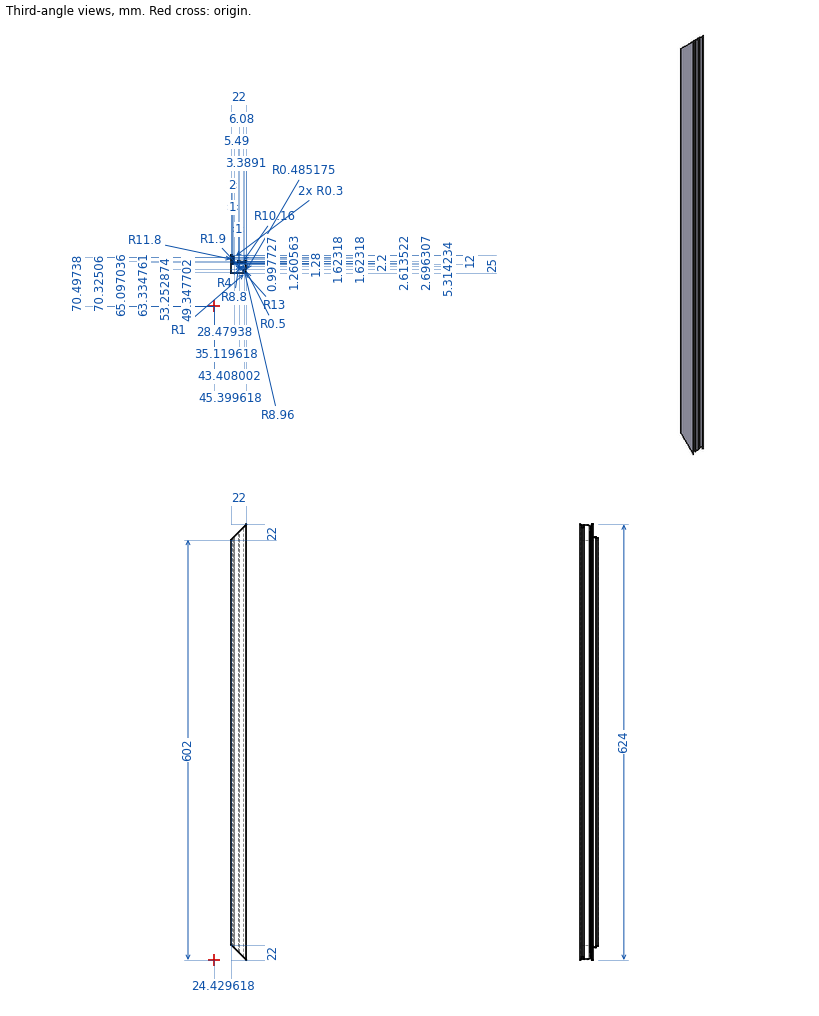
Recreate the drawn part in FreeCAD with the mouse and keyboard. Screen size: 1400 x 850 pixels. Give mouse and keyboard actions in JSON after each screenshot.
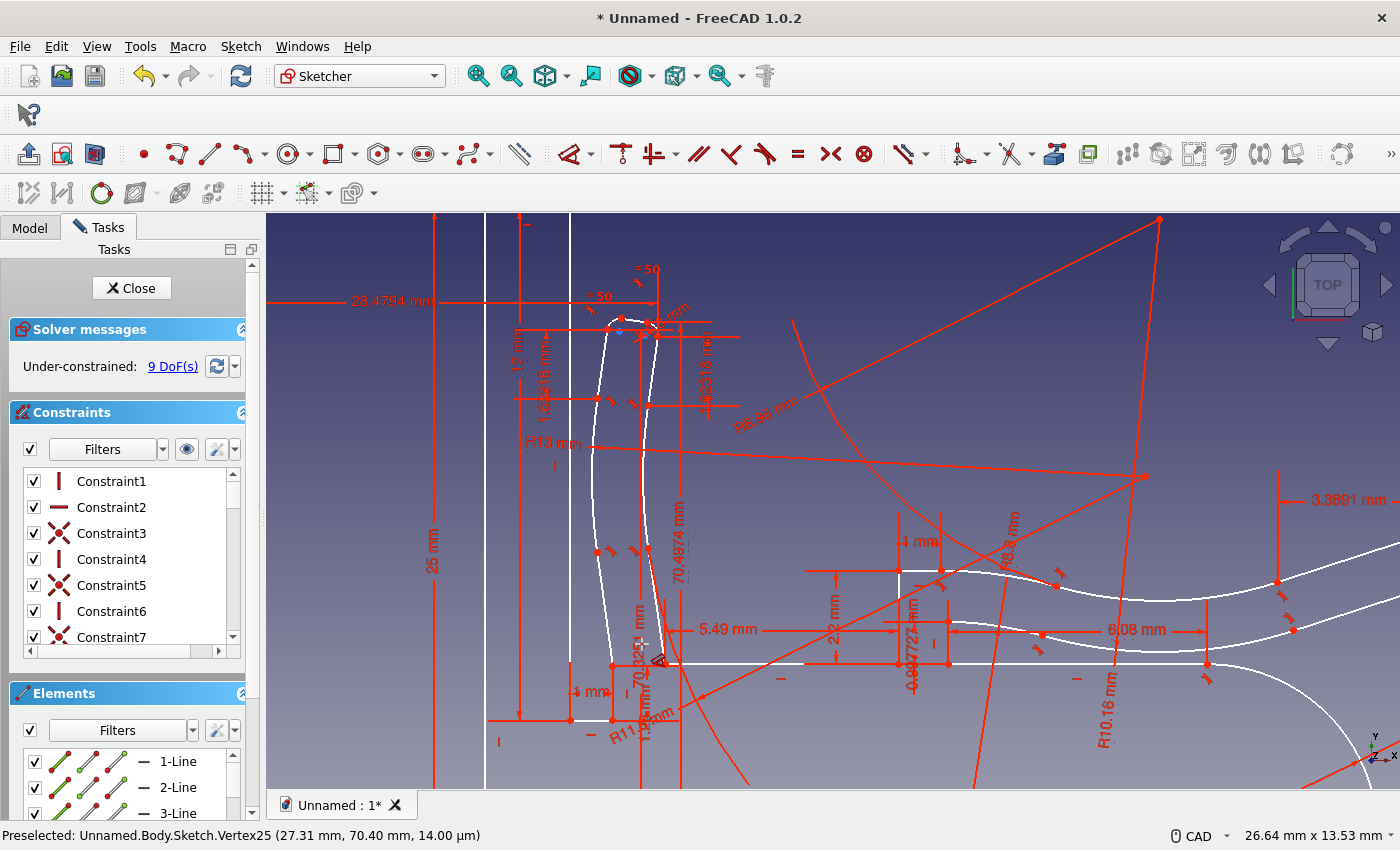
{"action": "left_click", "coordinate": [660, 630]}
{"action": "left_click", "coordinate": [614, 580]}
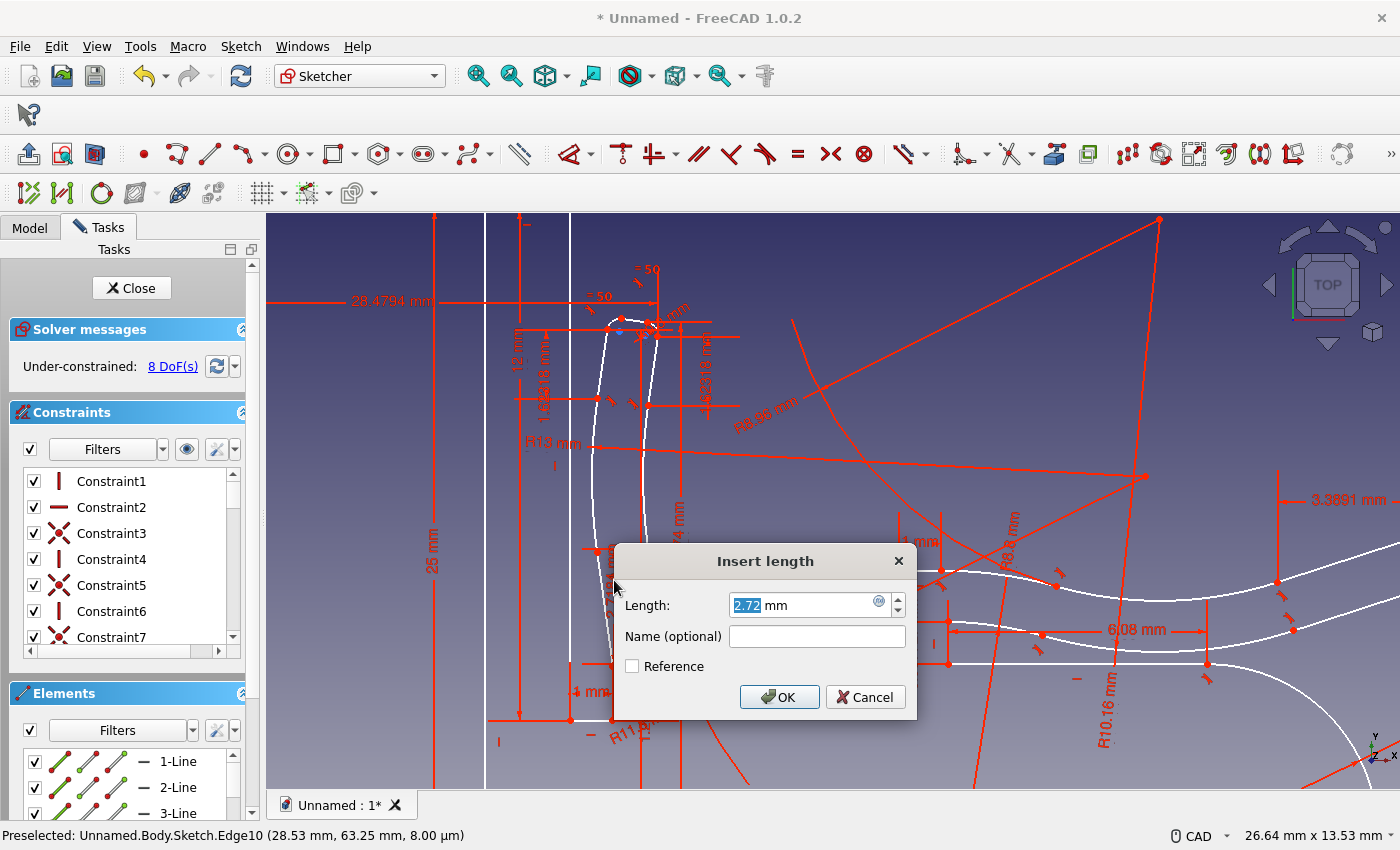
{"action": "type", "text": "2.696307"}
{"action": "key", "text": "Return"}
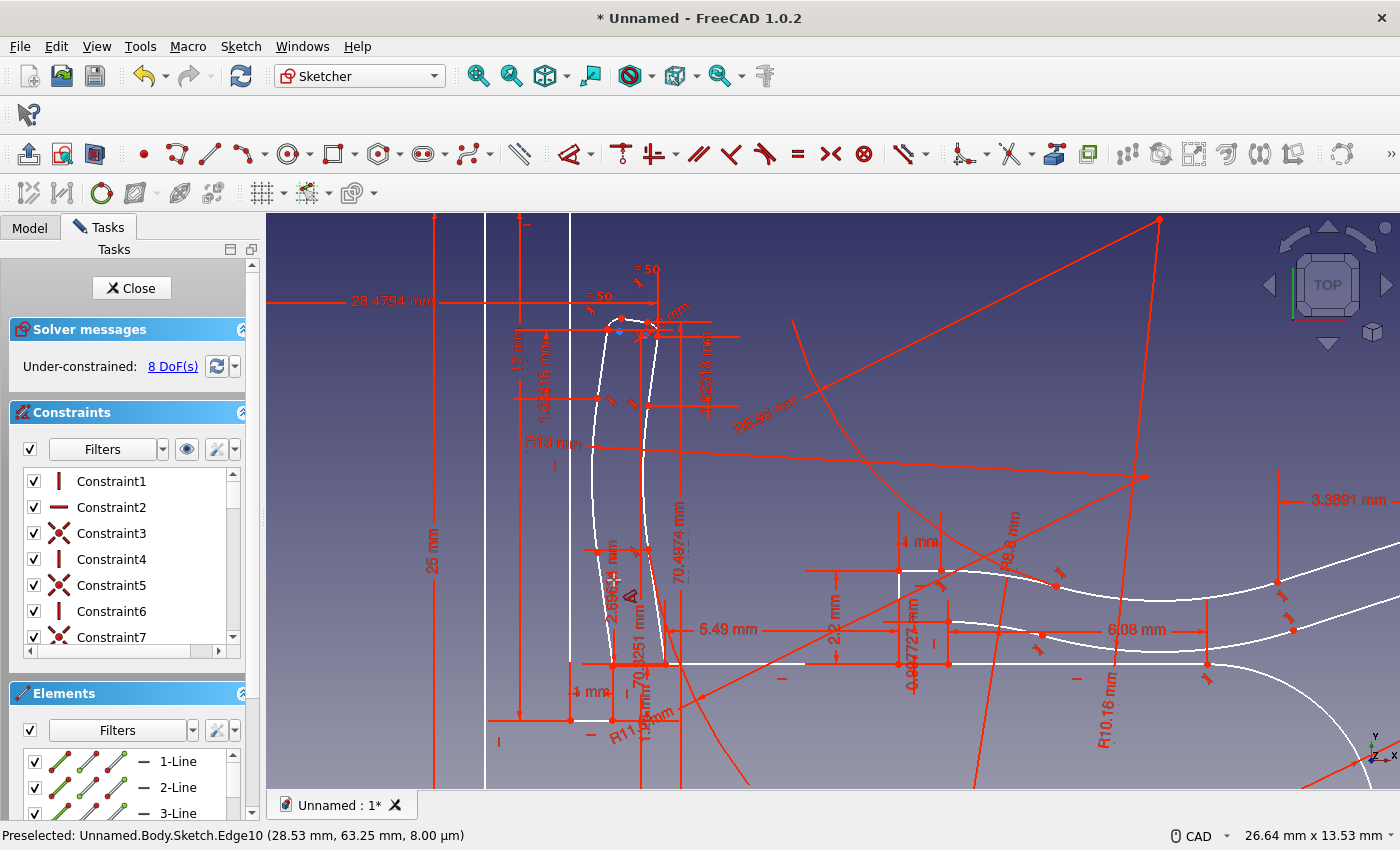
{"action": "left_click", "coordinate": [602, 586]}
{"action": "left_click", "coordinate": [539, 609]}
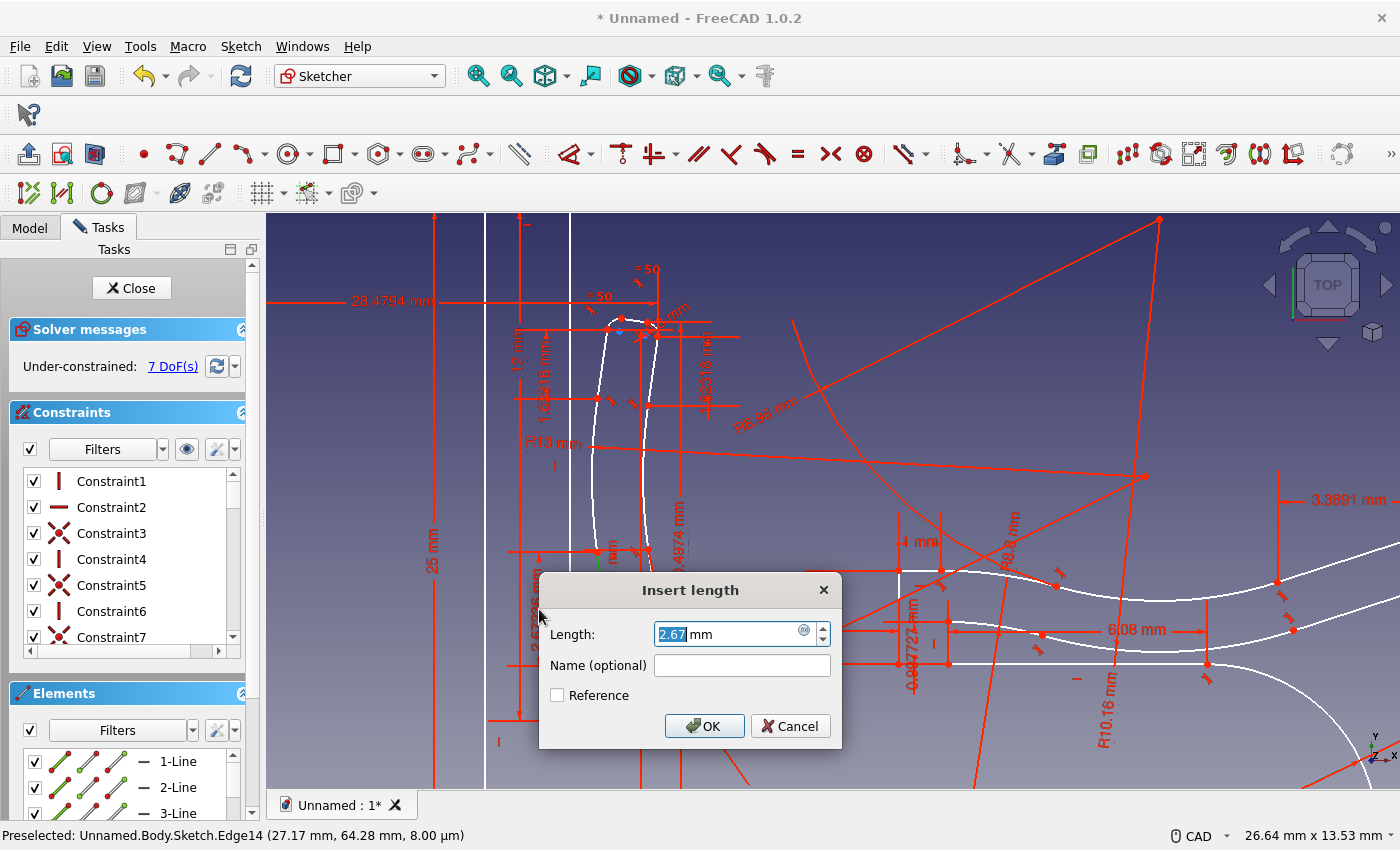
{"action": "type", "text": "2.613522"}
{"action": "key", "text": "Return"}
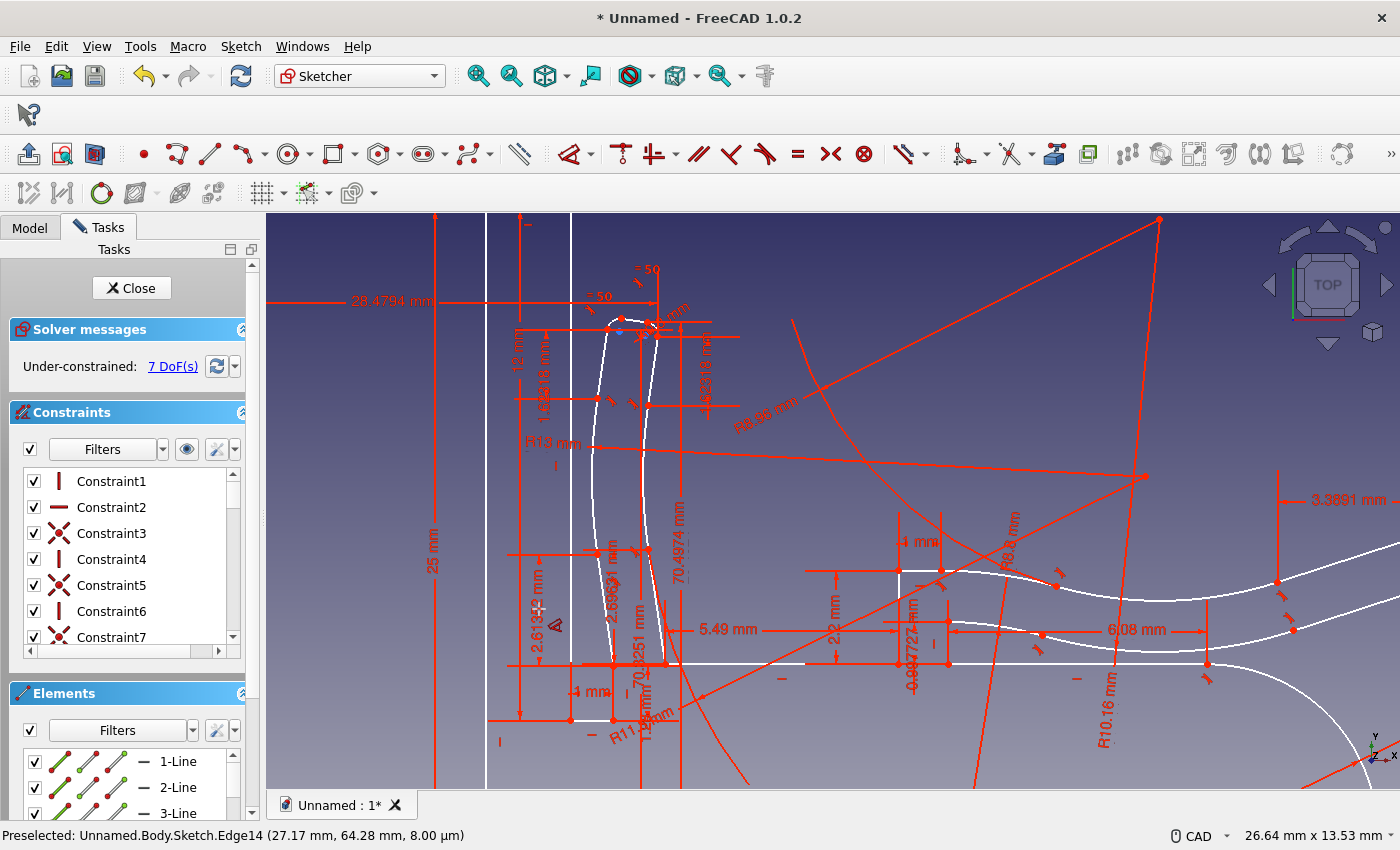
{"action": "scroll", "coordinate": [654, 362], "scroll_direction": "down", "scroll_amount": 5}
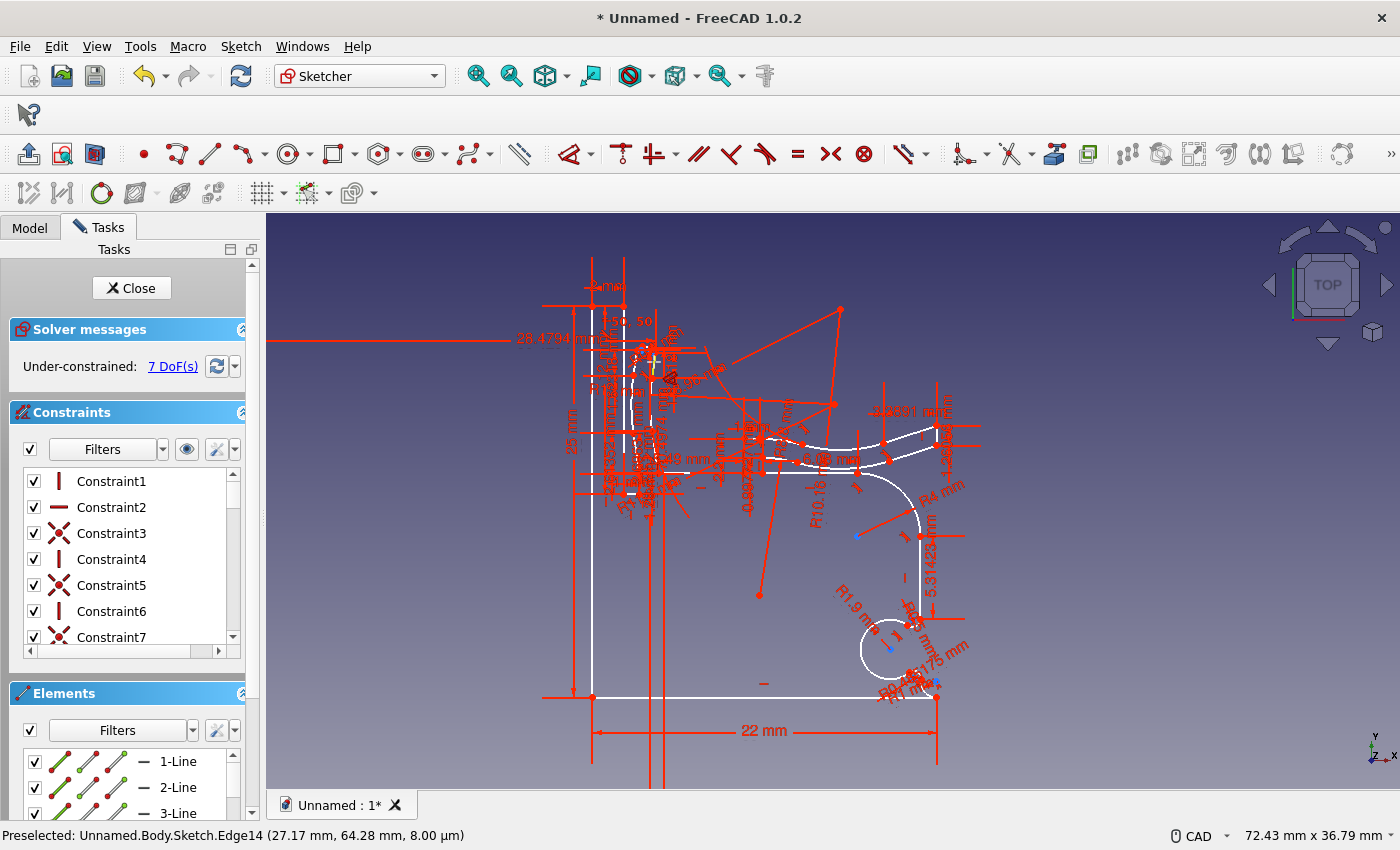
{"action": "scroll", "coordinate": [920, 619], "scroll_direction": "up", "scroll_amount": 3}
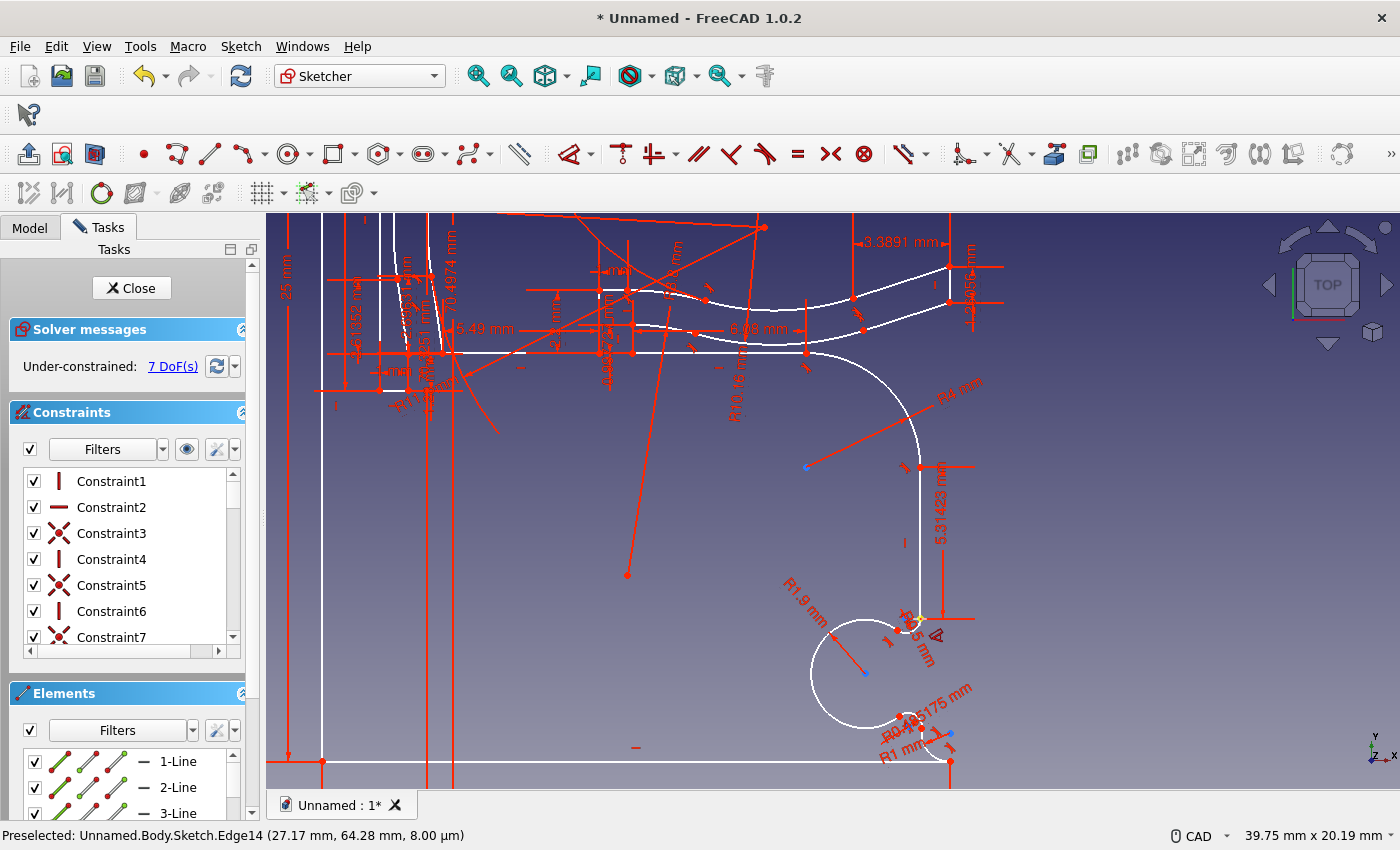
{"action": "left_click", "coordinate": [920, 619]}
{"action": "left_click", "coordinate": [607, 585]}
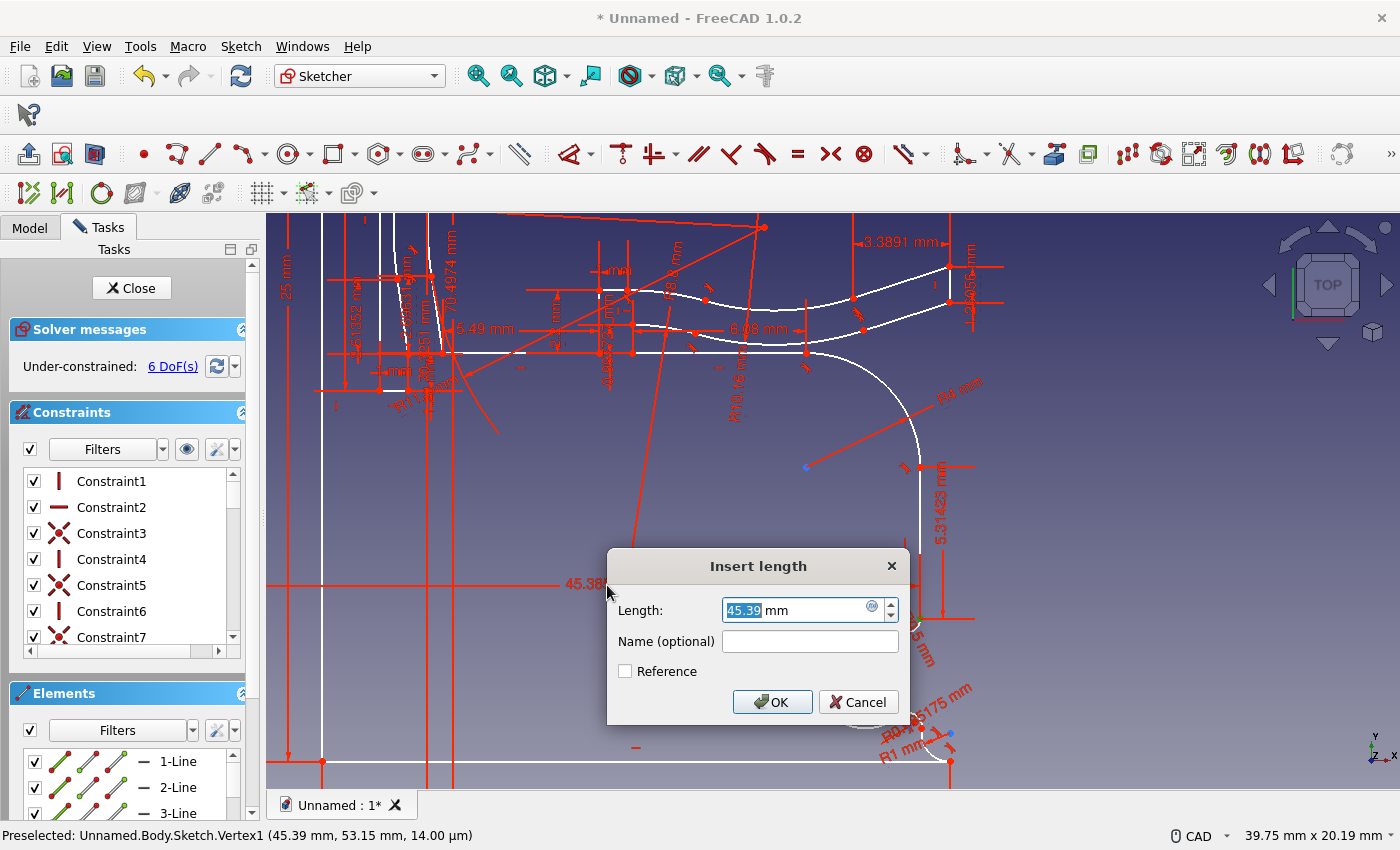
{"action": "type", "text": "45.399618"}
{"action": "key", "text": "Return"}